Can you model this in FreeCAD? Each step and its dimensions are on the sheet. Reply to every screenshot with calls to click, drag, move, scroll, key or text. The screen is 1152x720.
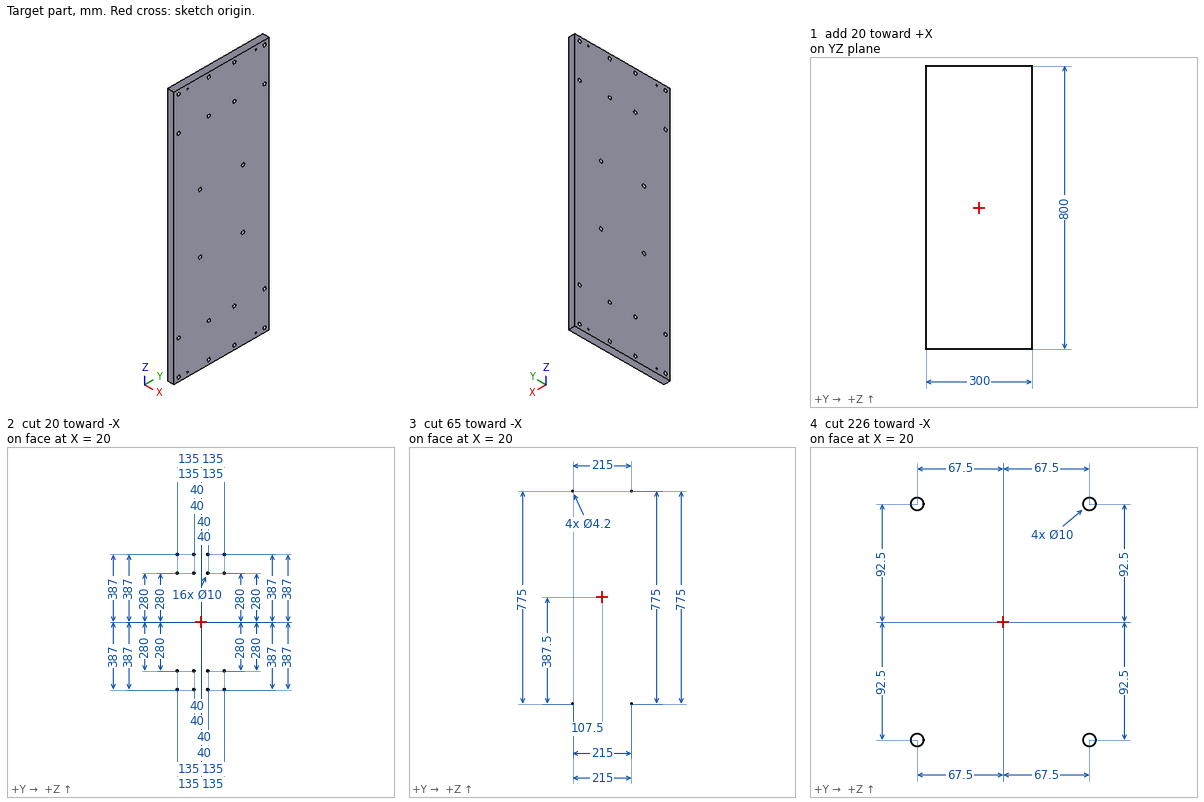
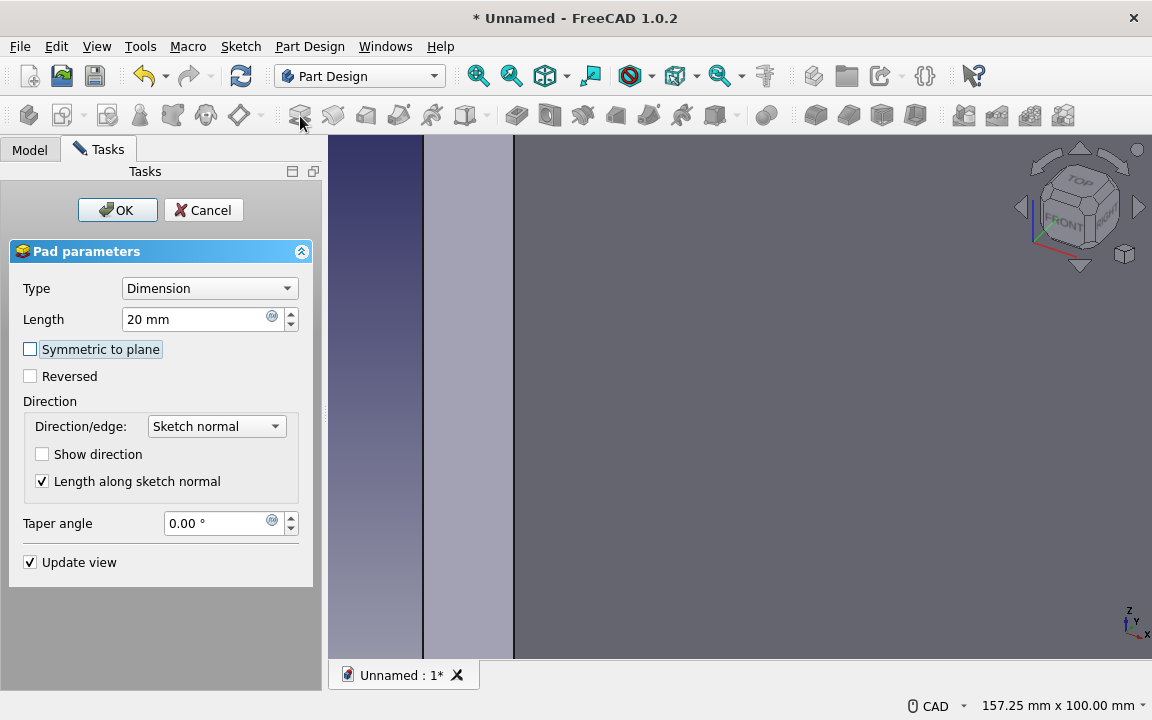
click(118, 210)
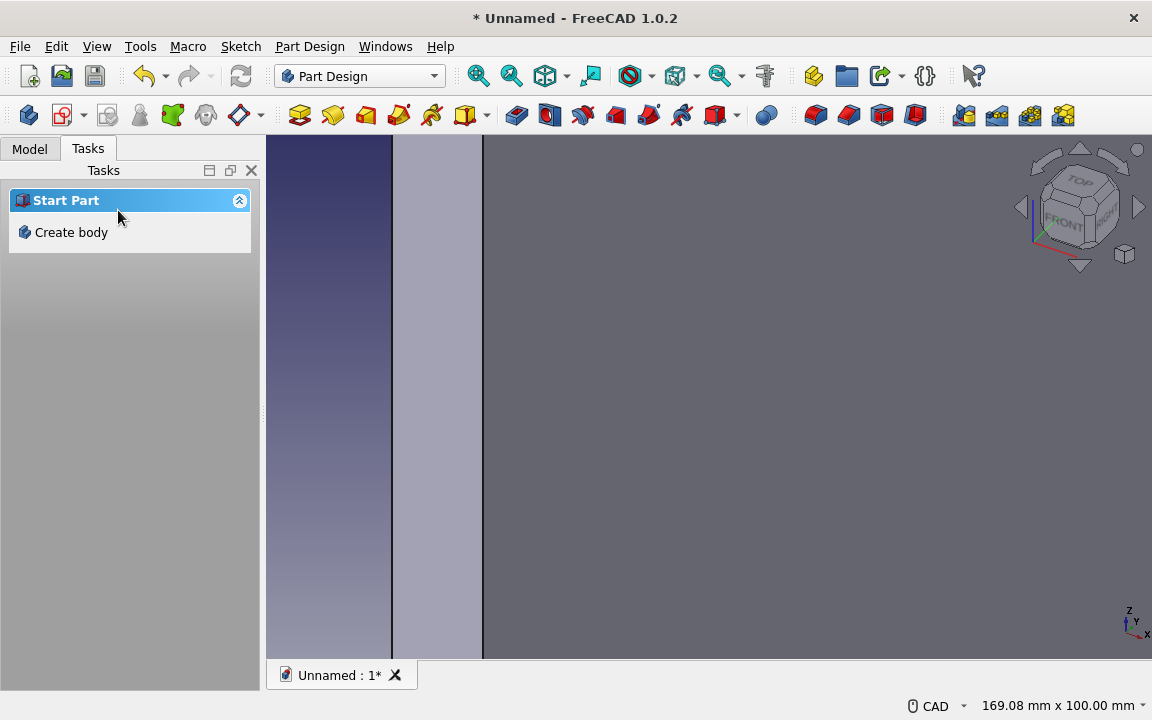
key(v)
key(f)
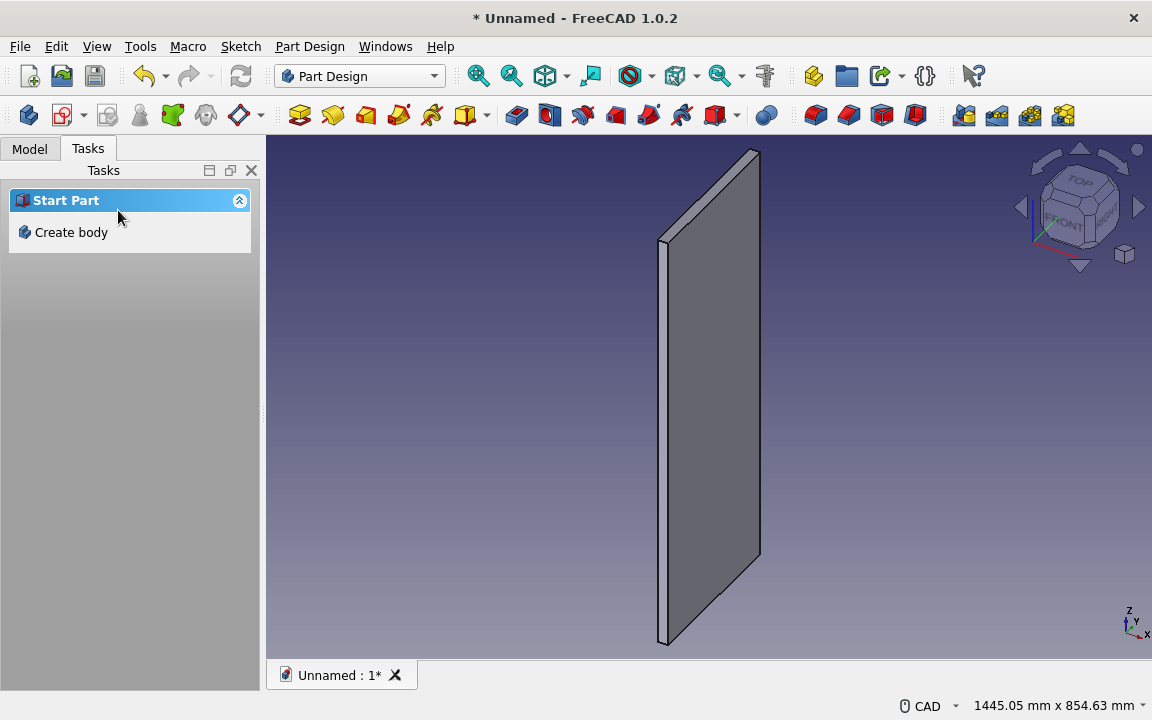
click(714, 398)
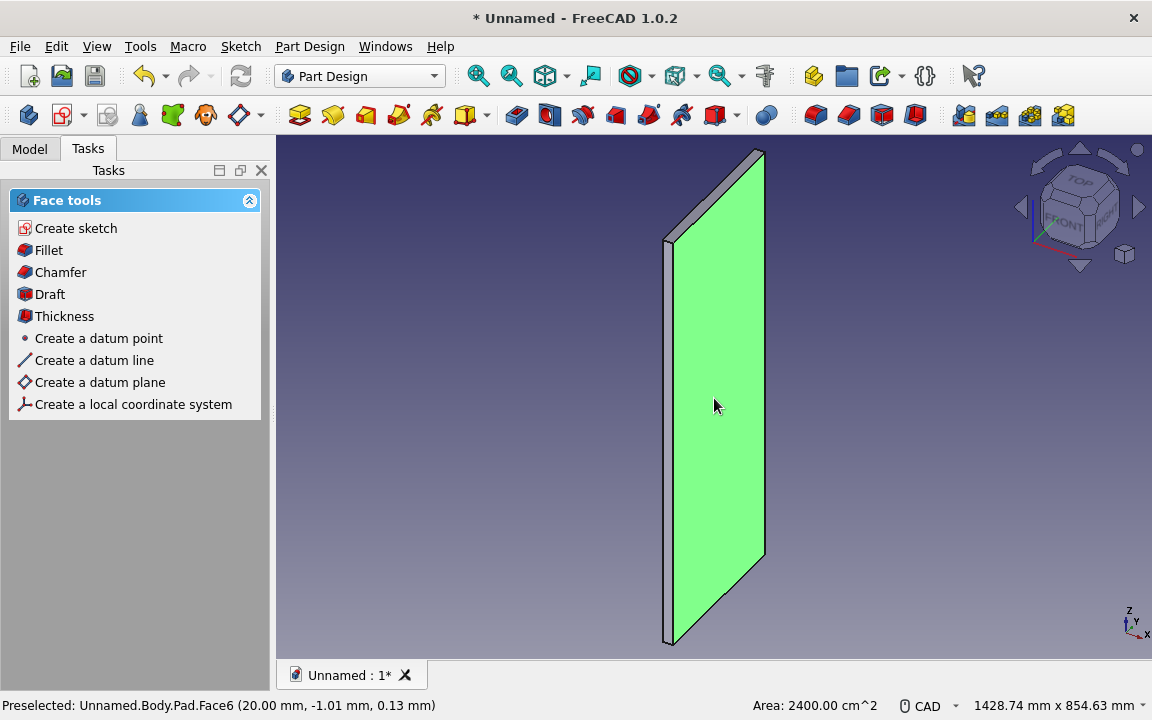
click(62, 116)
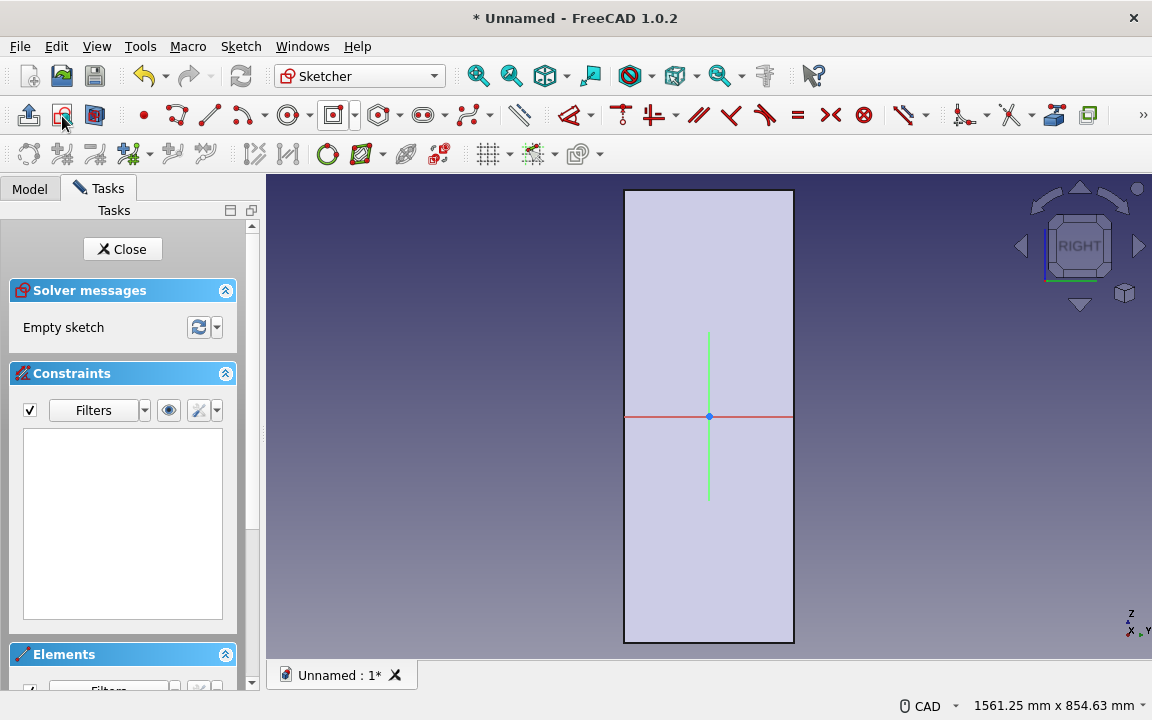
scroll(501, 416, down, 2)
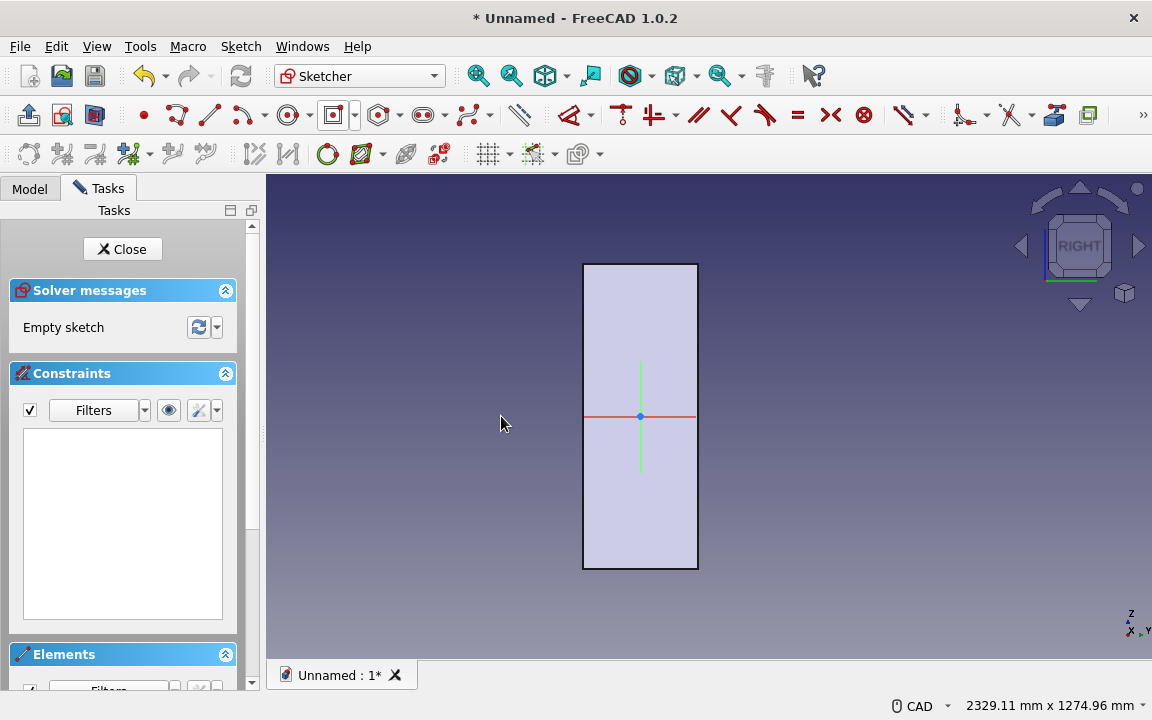
click(288, 116)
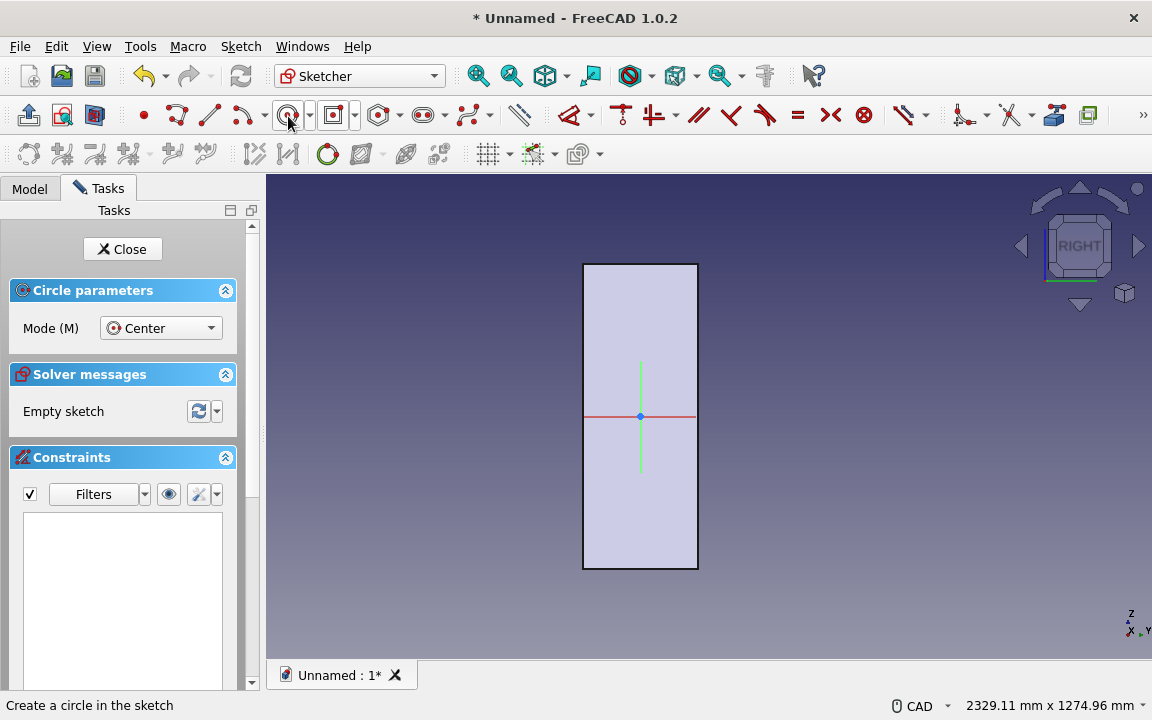
scroll(692, 269, up, 13)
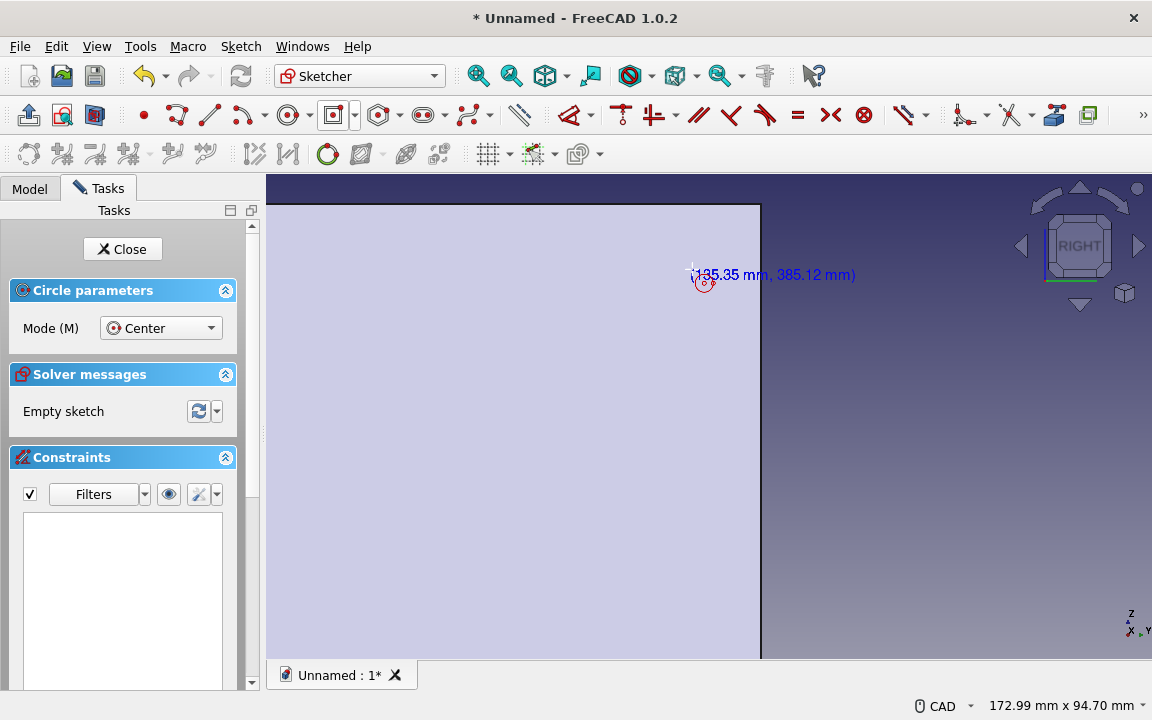
scroll(692, 269, down, 13)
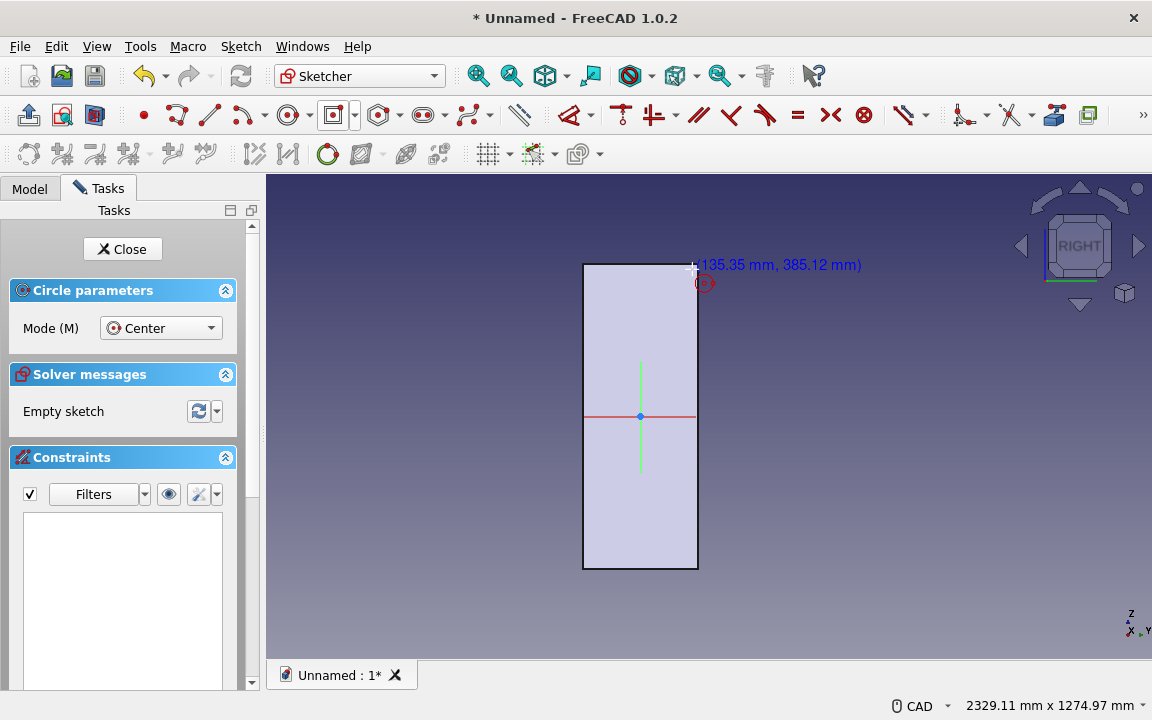
click(692, 269)
move(693, 268)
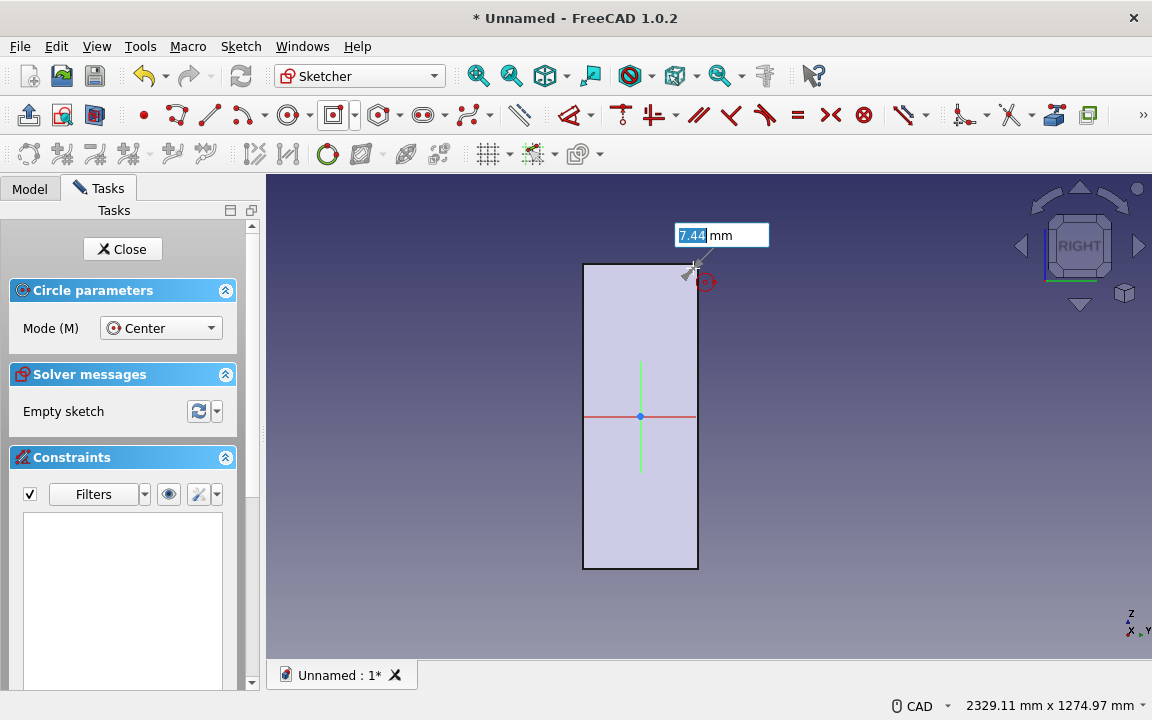
text(10)
key(Return)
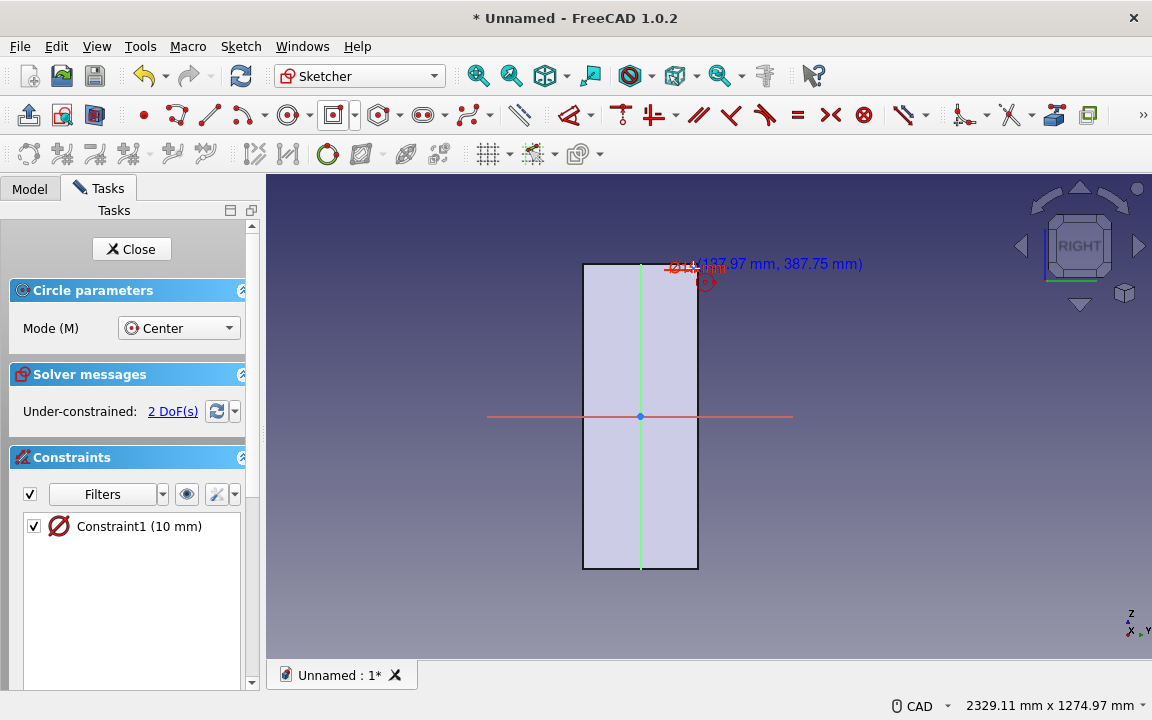
scroll(692, 310, up, 13)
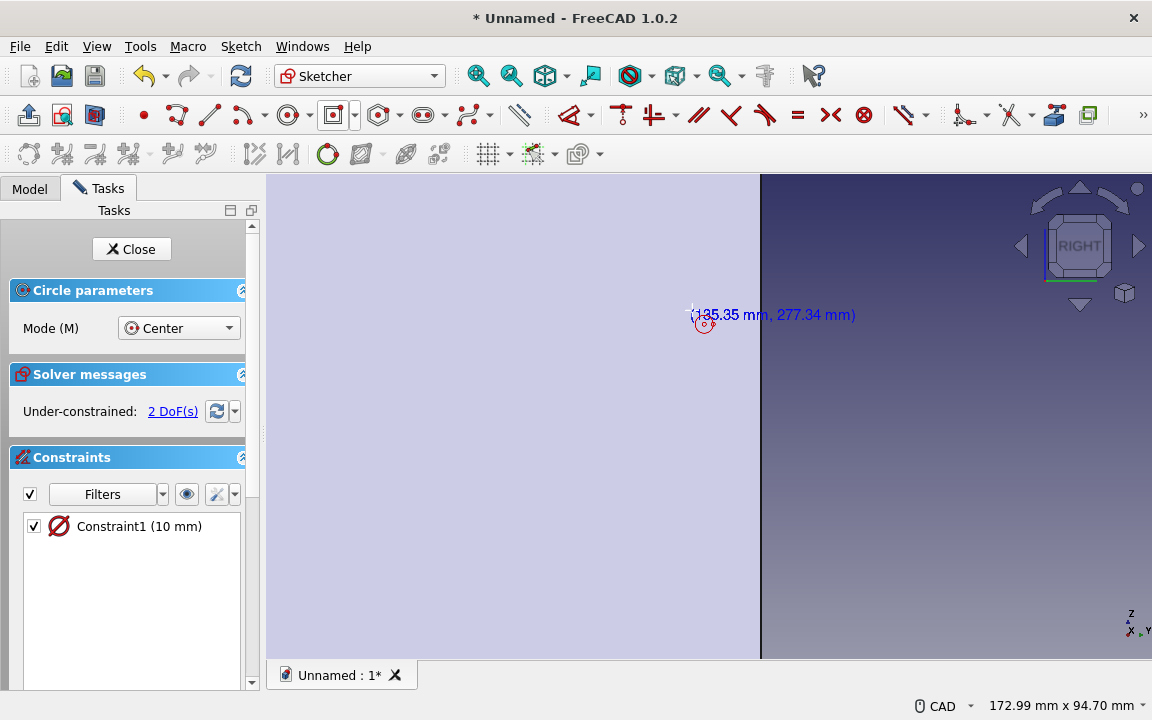
scroll(692, 310, down, 13)